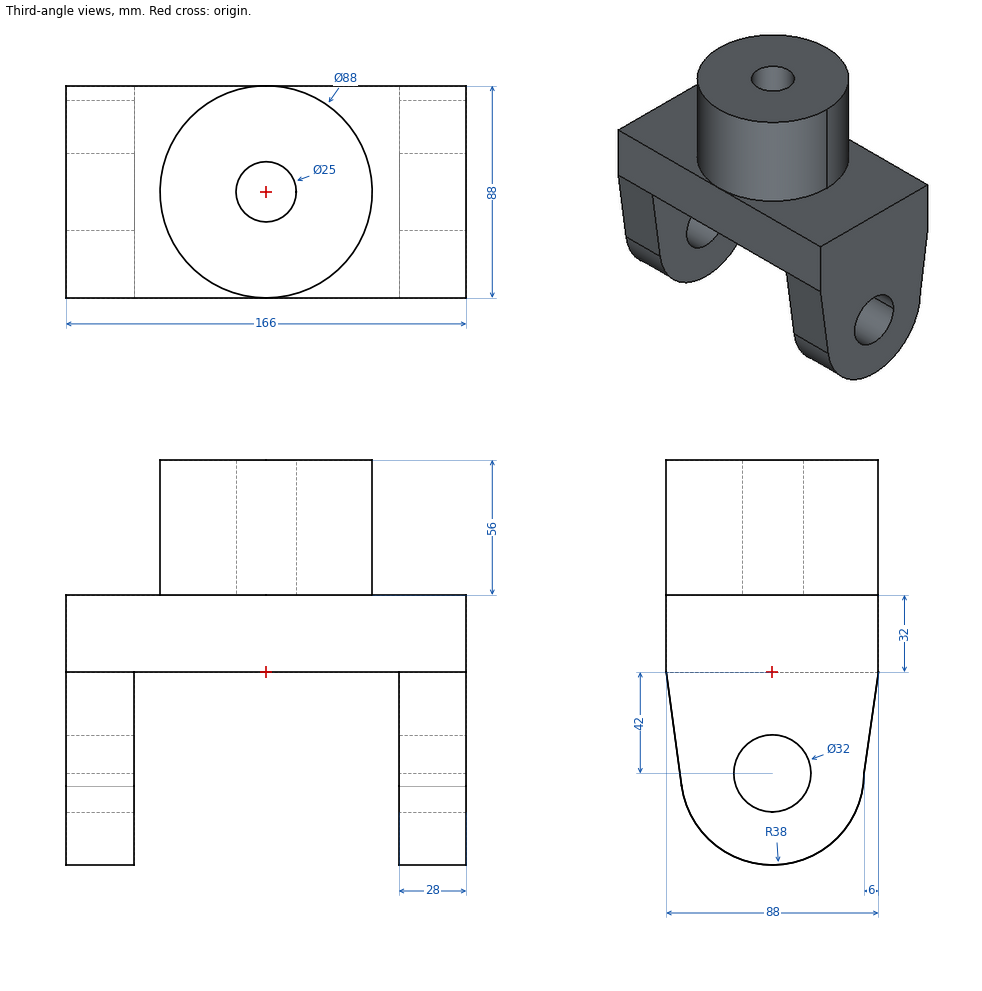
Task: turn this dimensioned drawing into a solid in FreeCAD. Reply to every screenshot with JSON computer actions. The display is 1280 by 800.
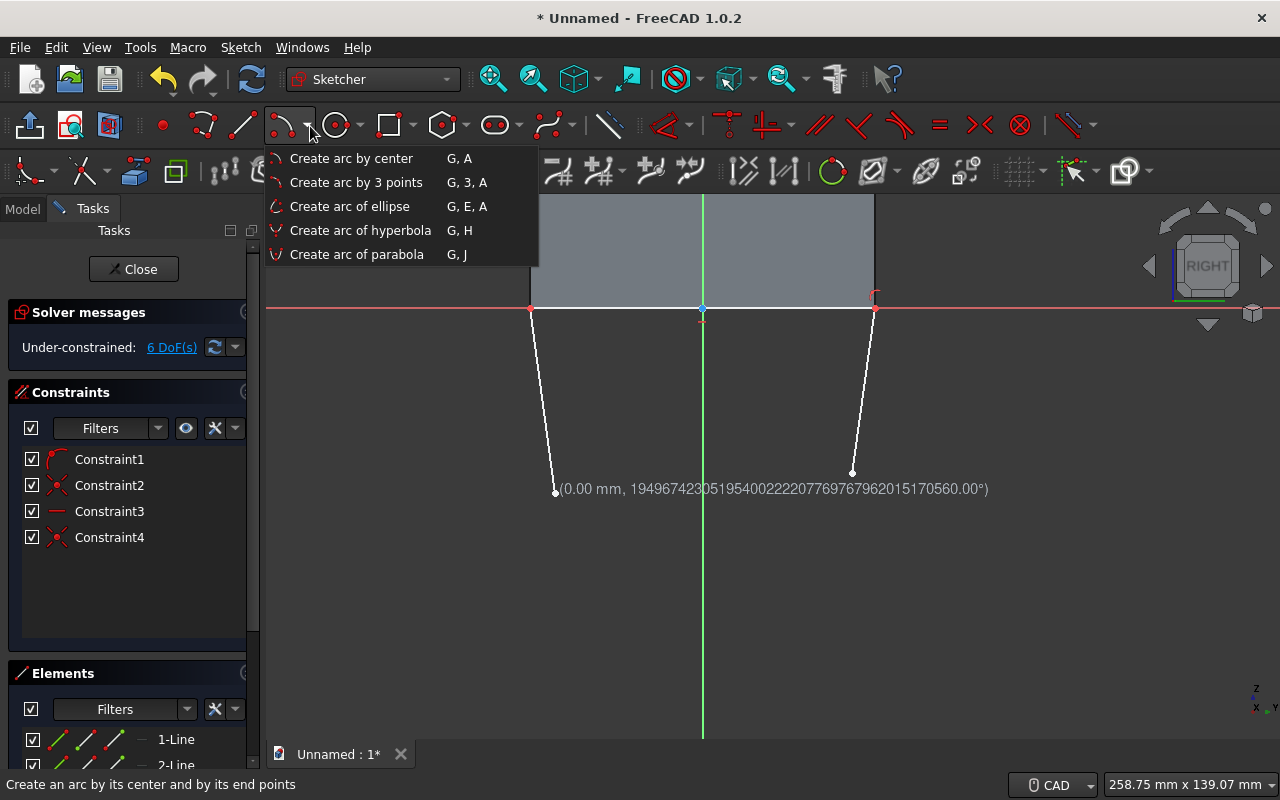
{"action": "left_click", "coordinate": [402, 182]}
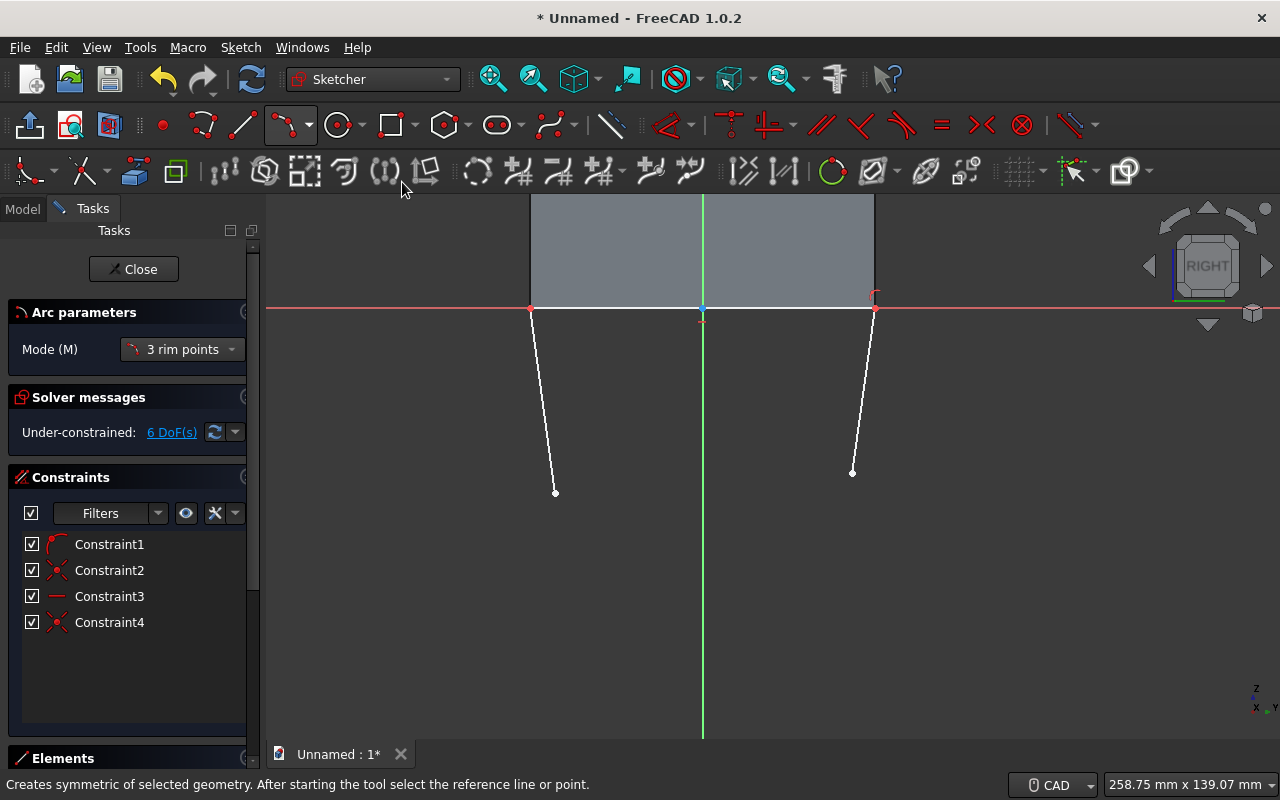
{"action": "left_click", "coordinate": [555, 494]}
{"action": "left_click", "coordinate": [852, 474]}
{"action": "left_click", "coordinate": [668, 618]}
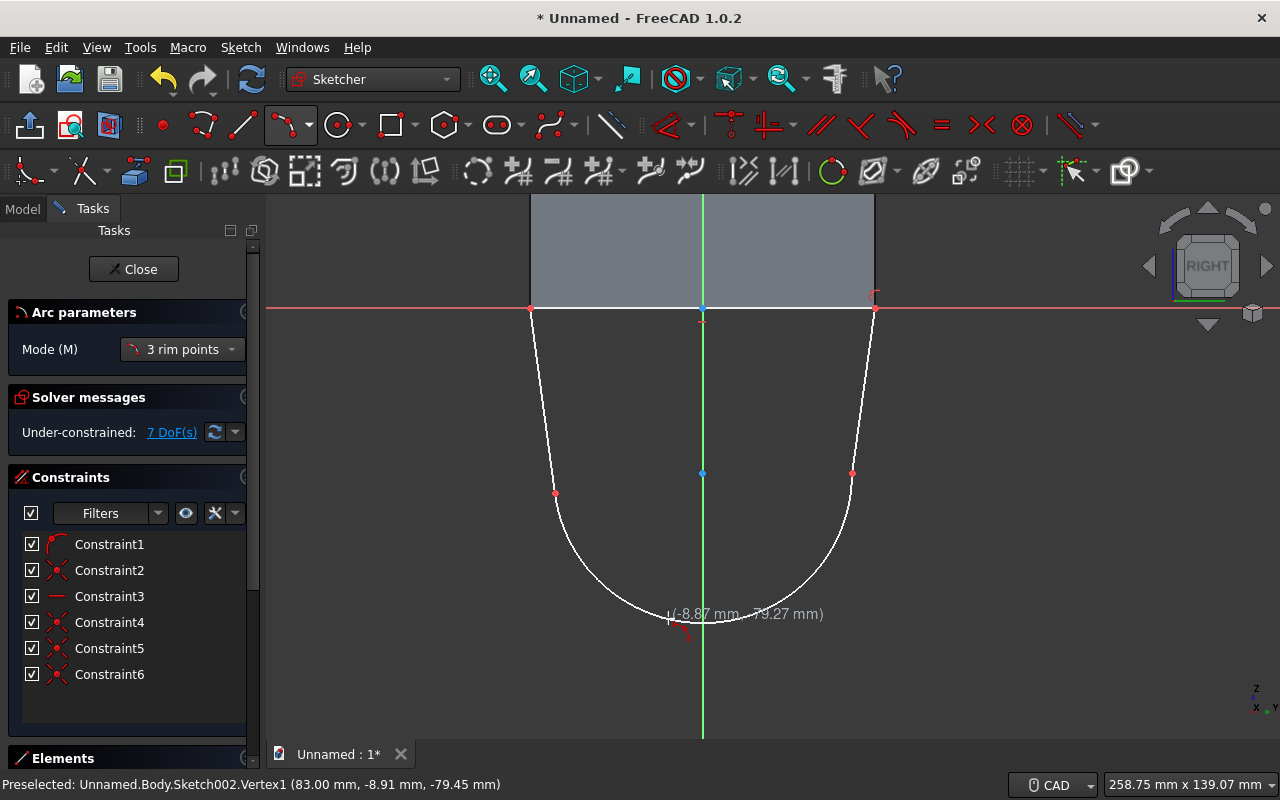
{"action": "left_click", "coordinate": [338, 126]}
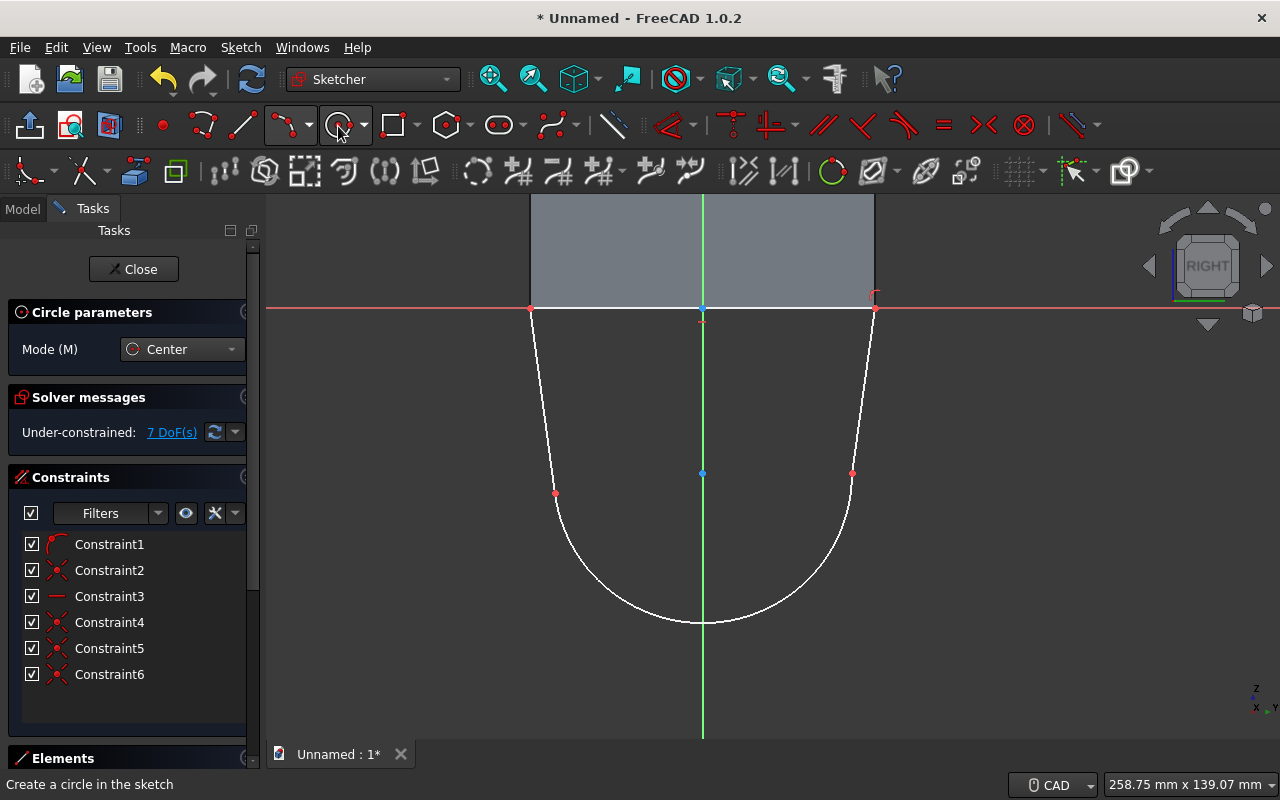
{"action": "left_click", "coordinate": [703, 473]}
{"action": "left_click", "coordinate": [747, 429]}
{"action": "key", "text": "Escape"}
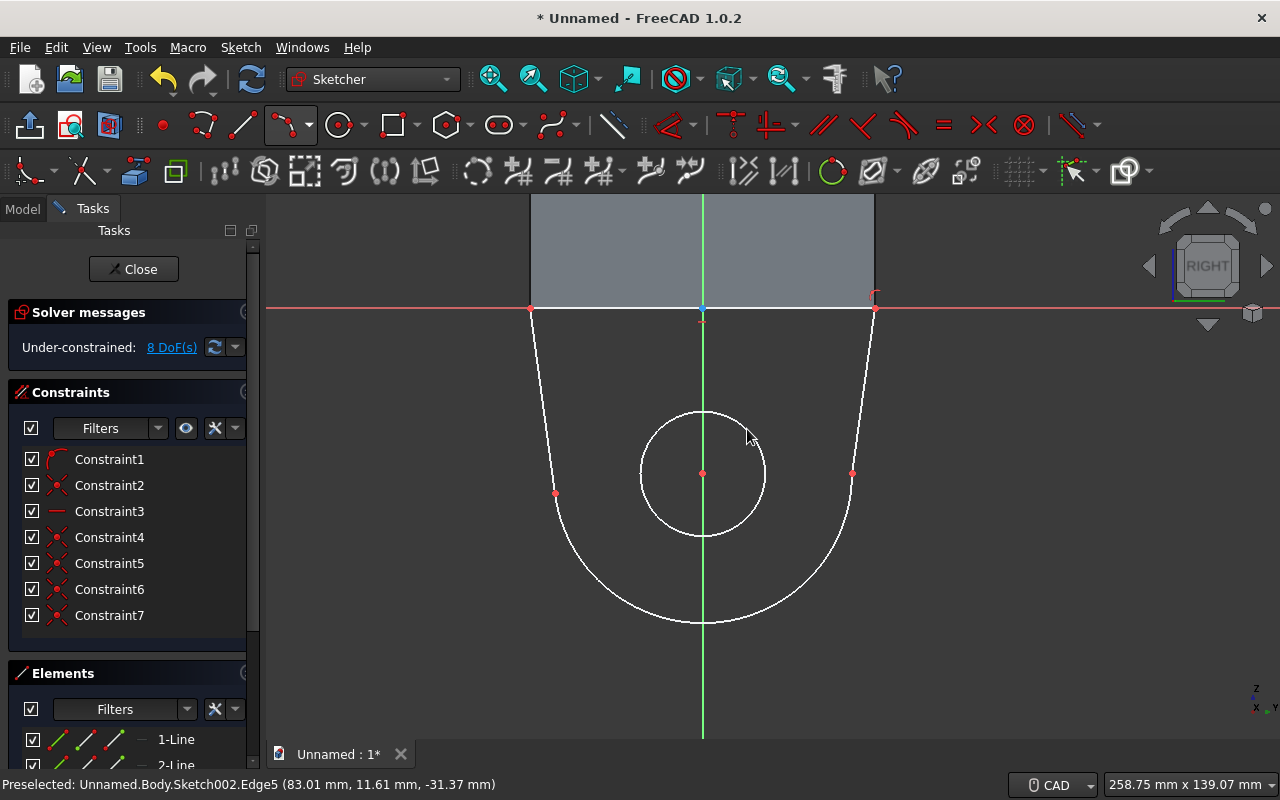
{"action": "left_click", "coordinate": [538, 364]}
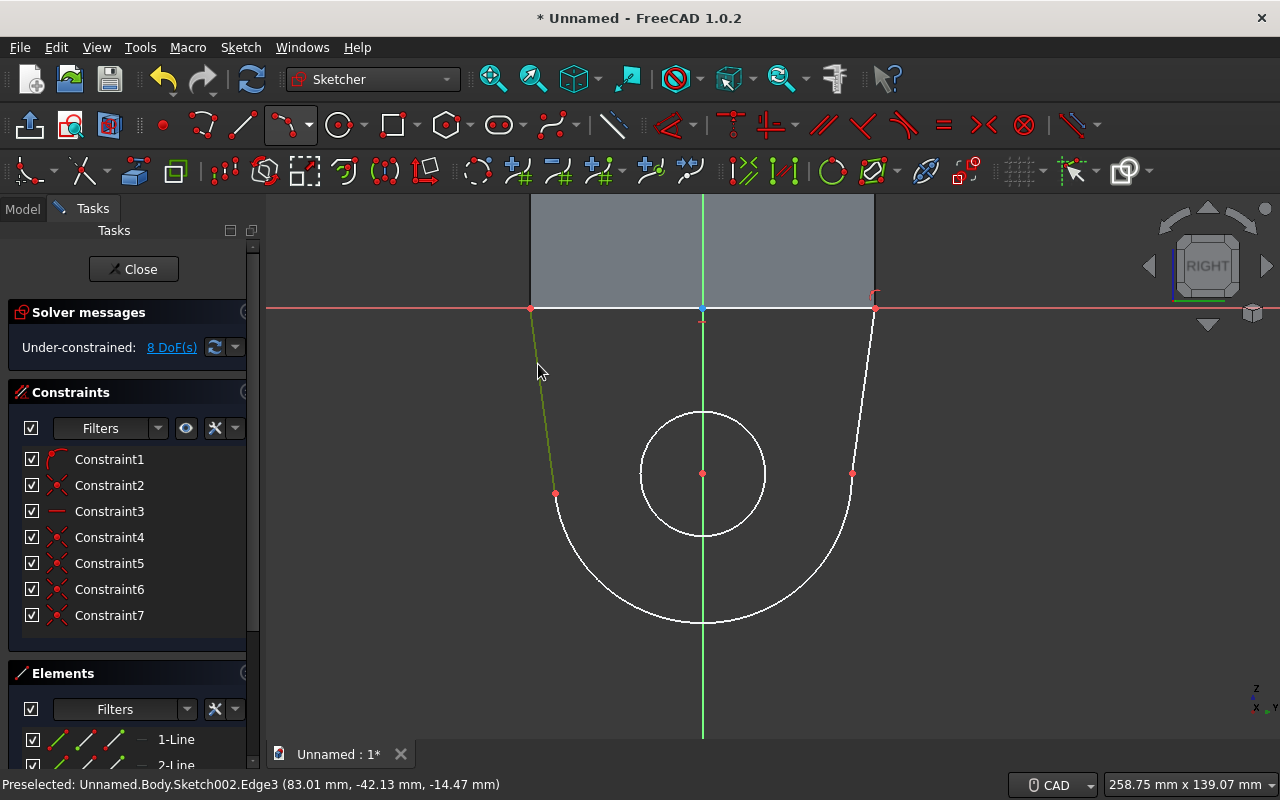
{"action": "left_click", "coordinate": [627, 602]}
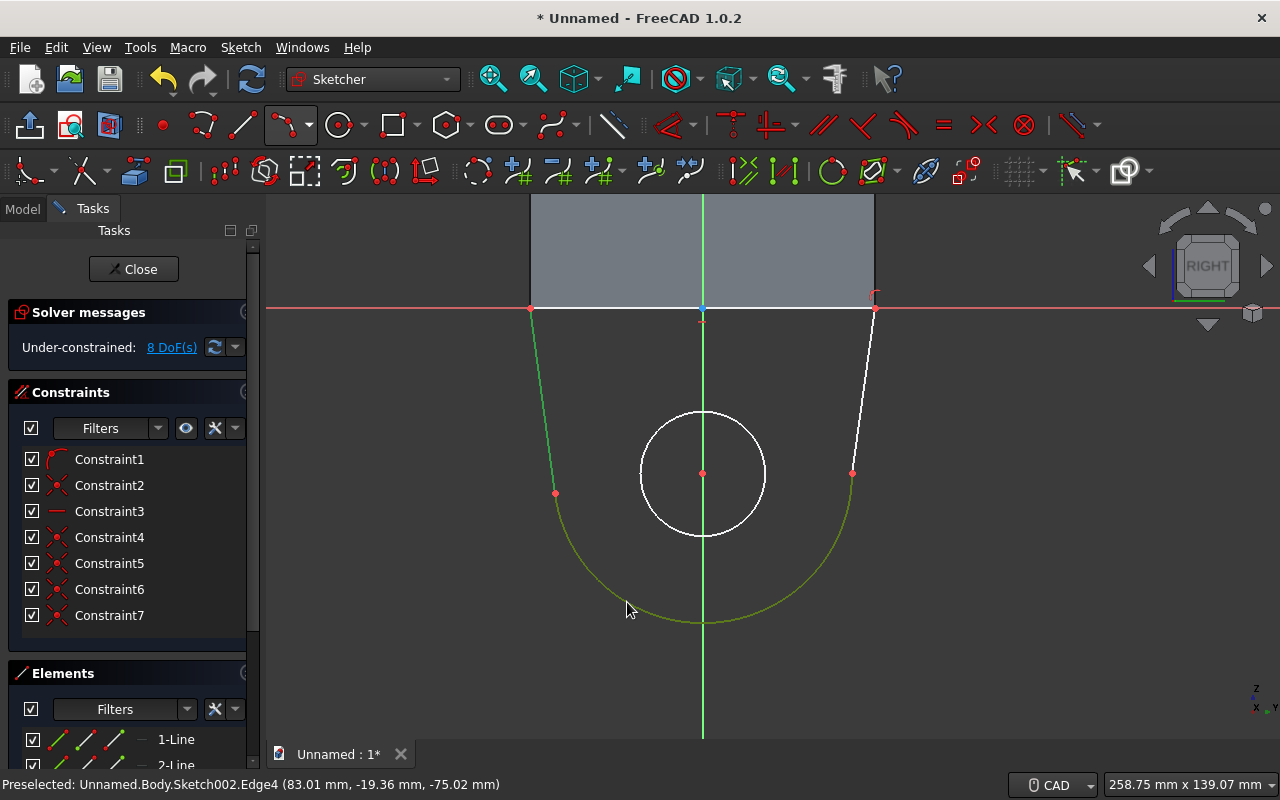
{"action": "left_click", "coordinate": [904, 126]}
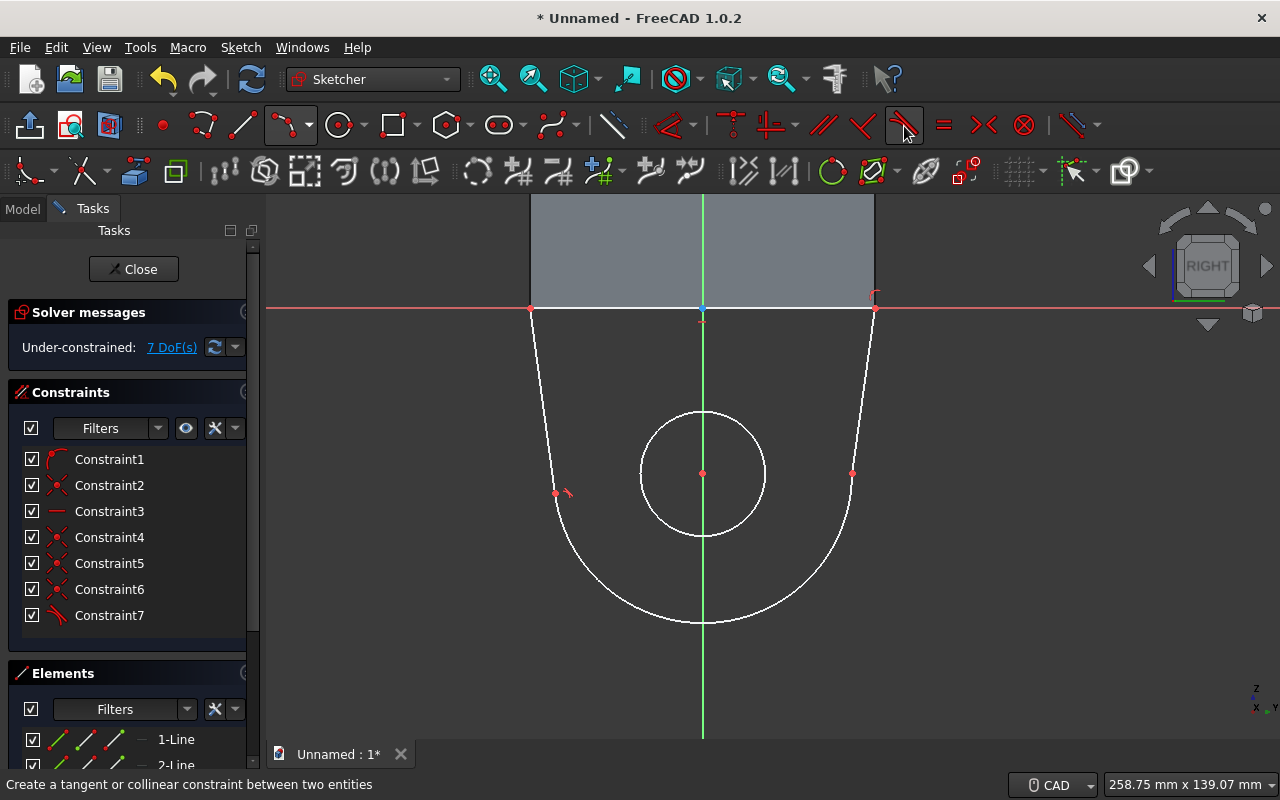
{"action": "left_click", "coordinate": [703, 474]}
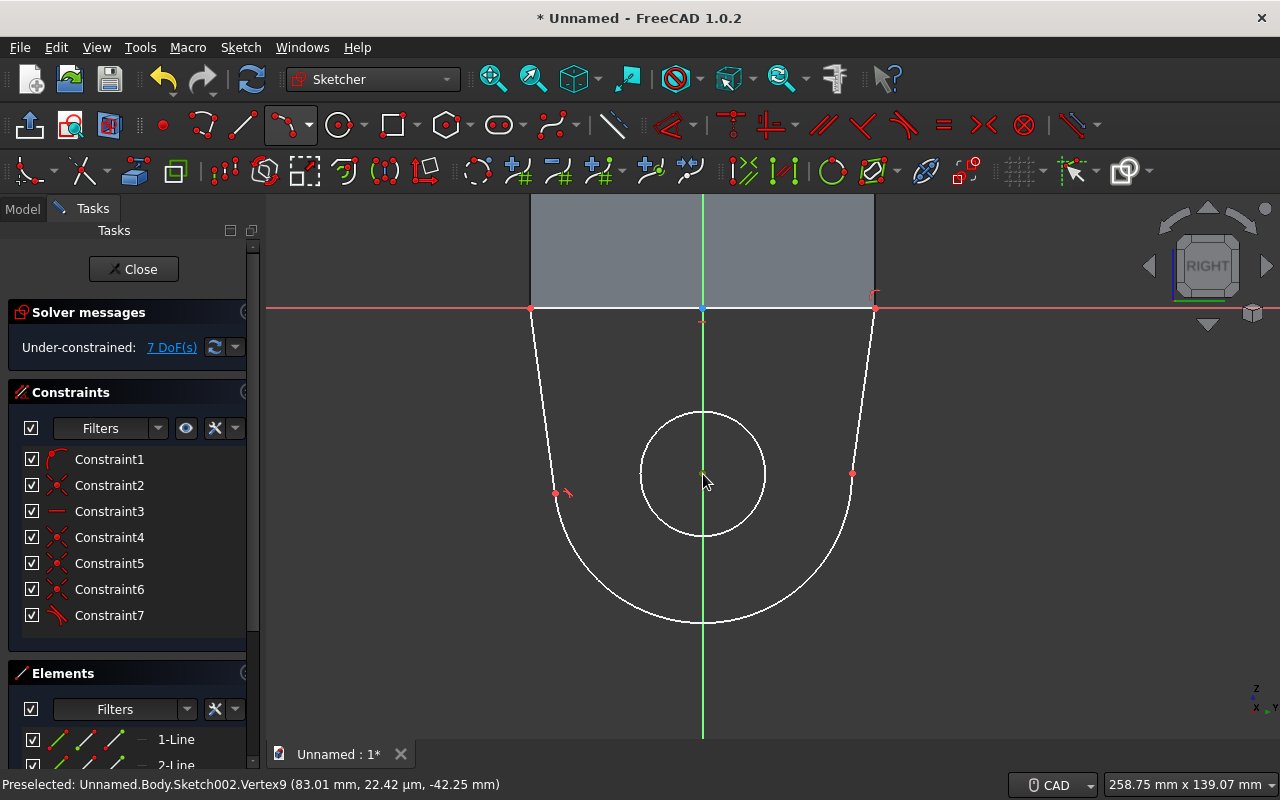
{"action": "left_click", "coordinate": [703, 676]}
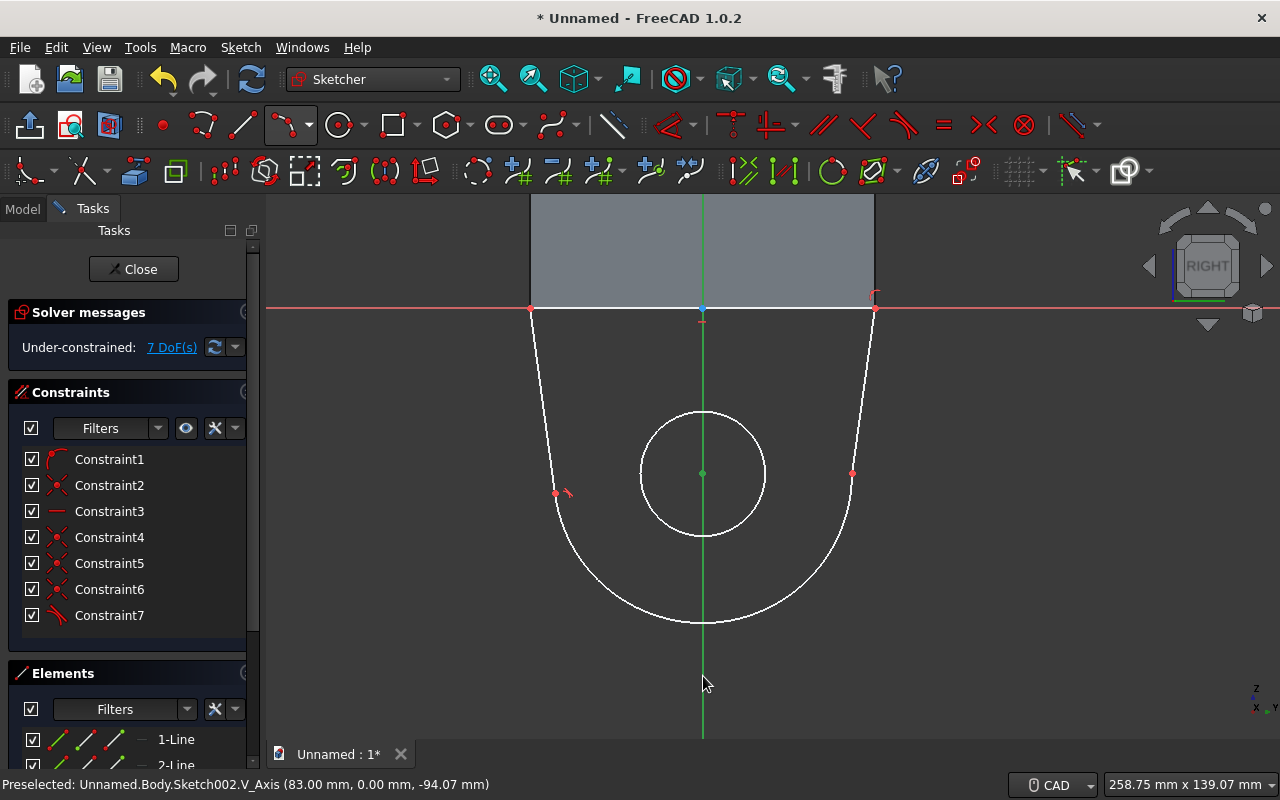
{"action": "left_click", "coordinate": [732, 126]}